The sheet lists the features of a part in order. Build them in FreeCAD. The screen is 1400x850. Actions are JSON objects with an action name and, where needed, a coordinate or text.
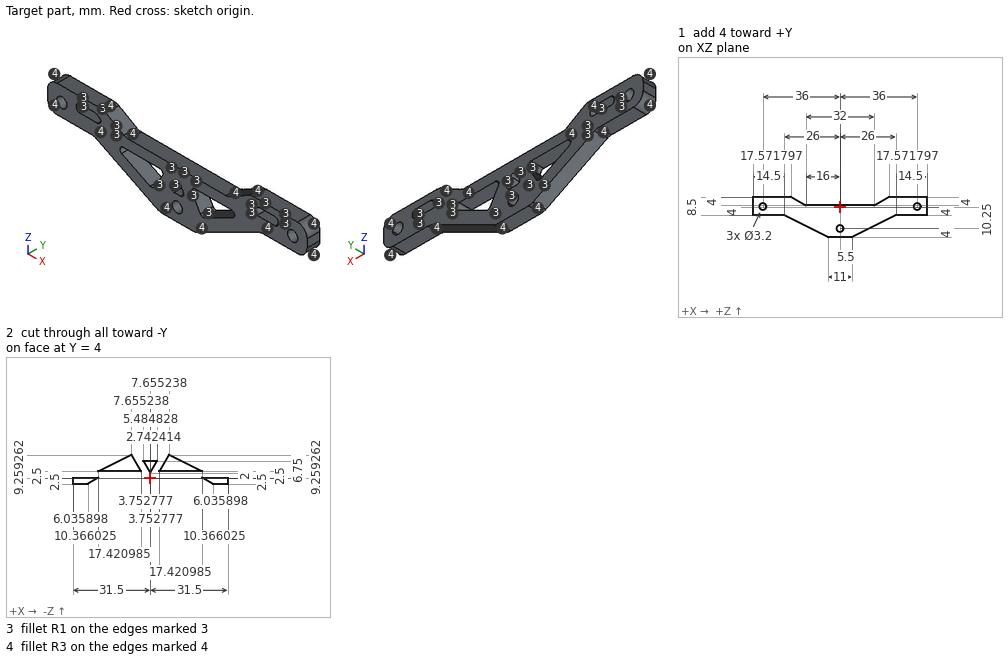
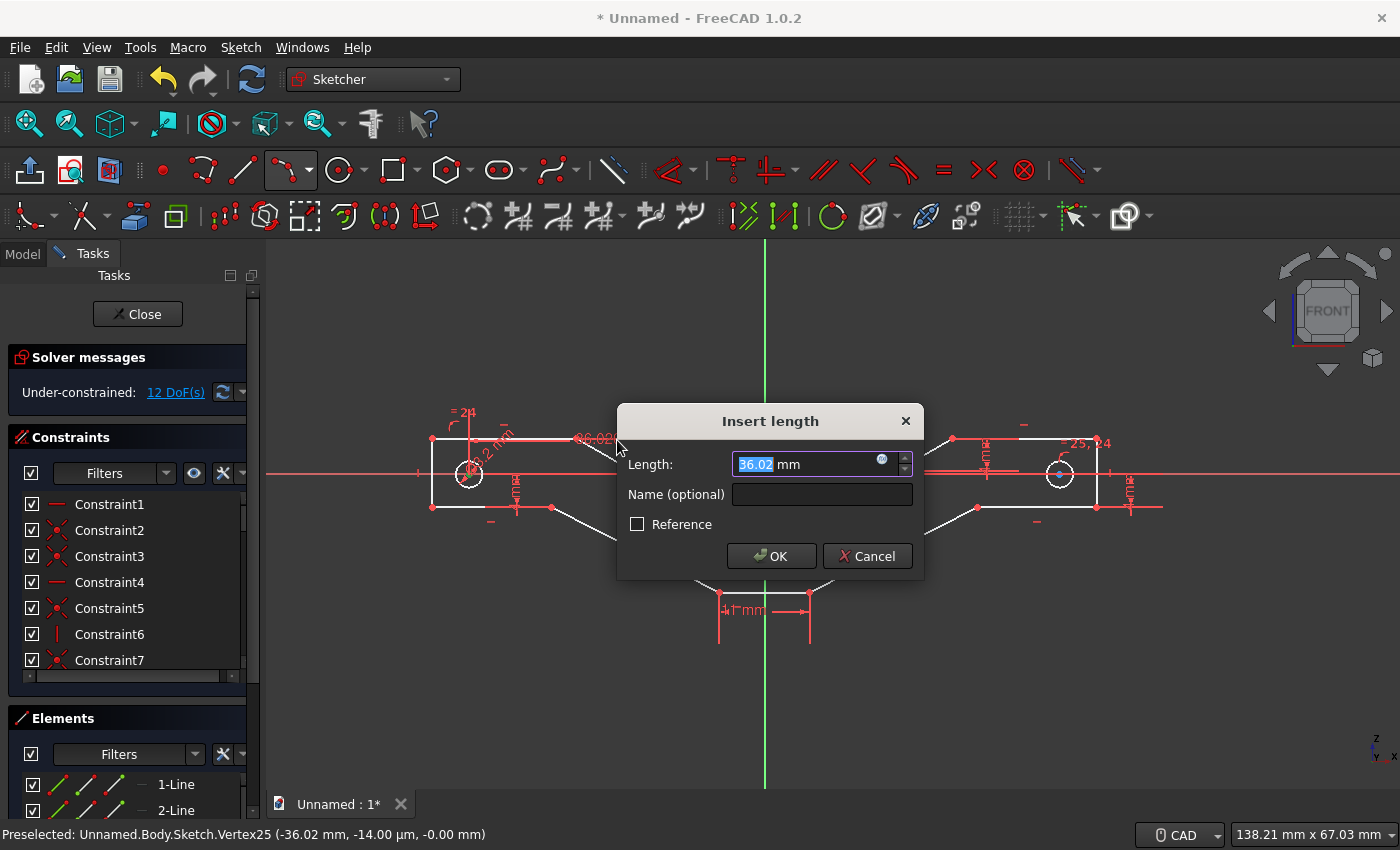
{"action": "type", "text": "36"}
{"action": "key", "text": "Return"}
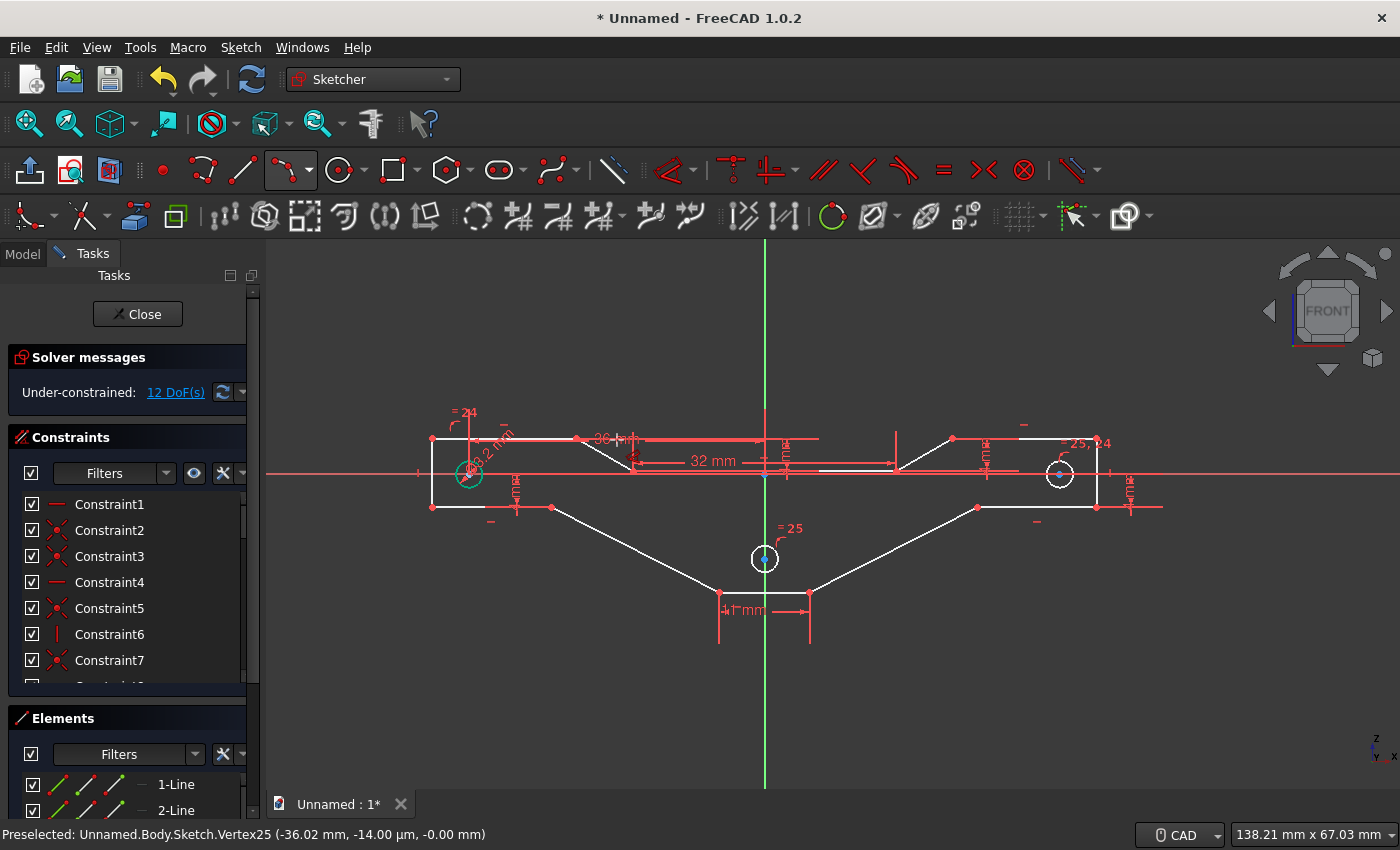
{"action": "left_click", "coordinate": [1060, 474]}
{"action": "left_click", "coordinate": [912, 440]}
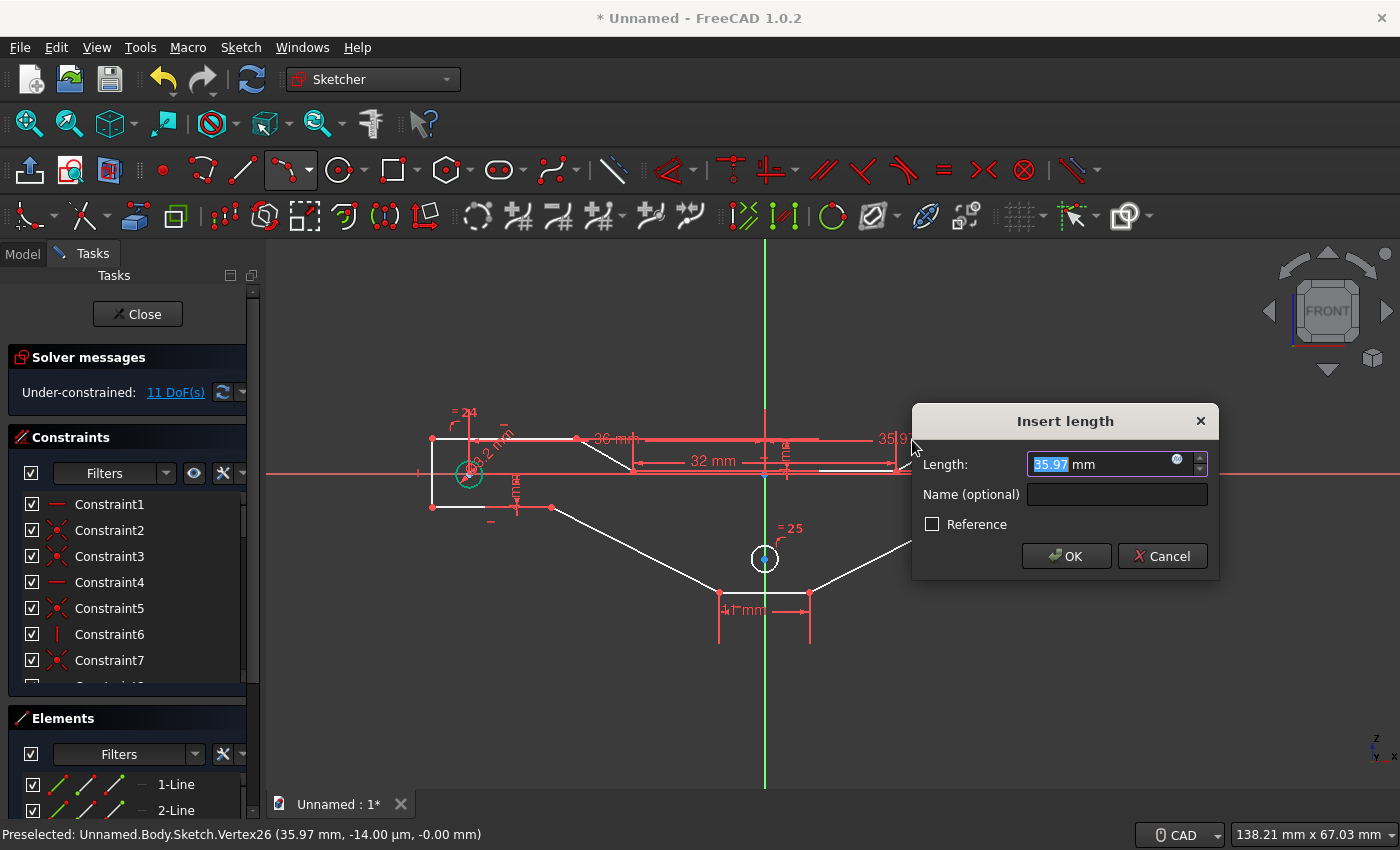
{"action": "type", "text": "36"}
{"action": "key", "text": "Return"}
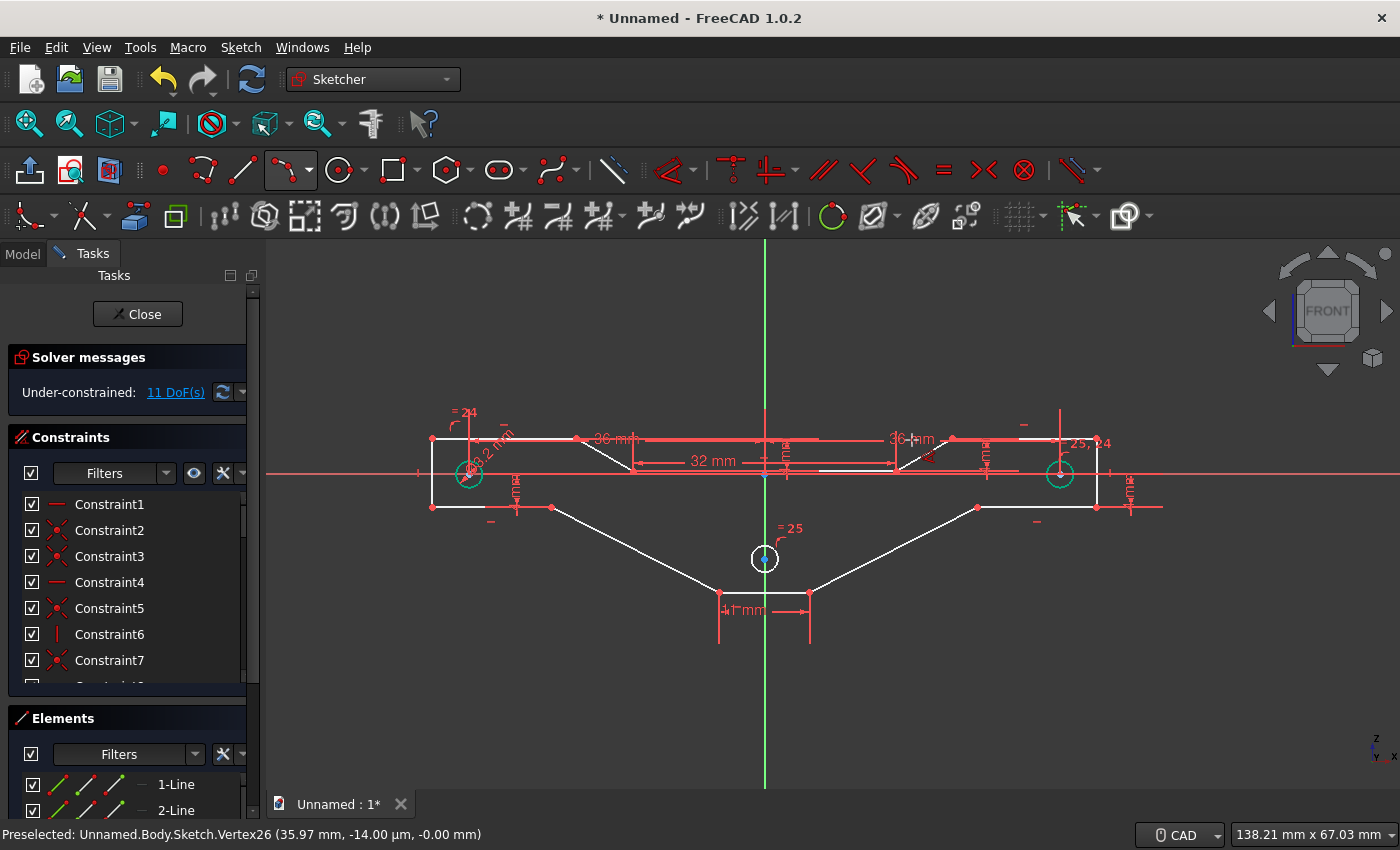
{"action": "left_click", "coordinate": [810, 593]}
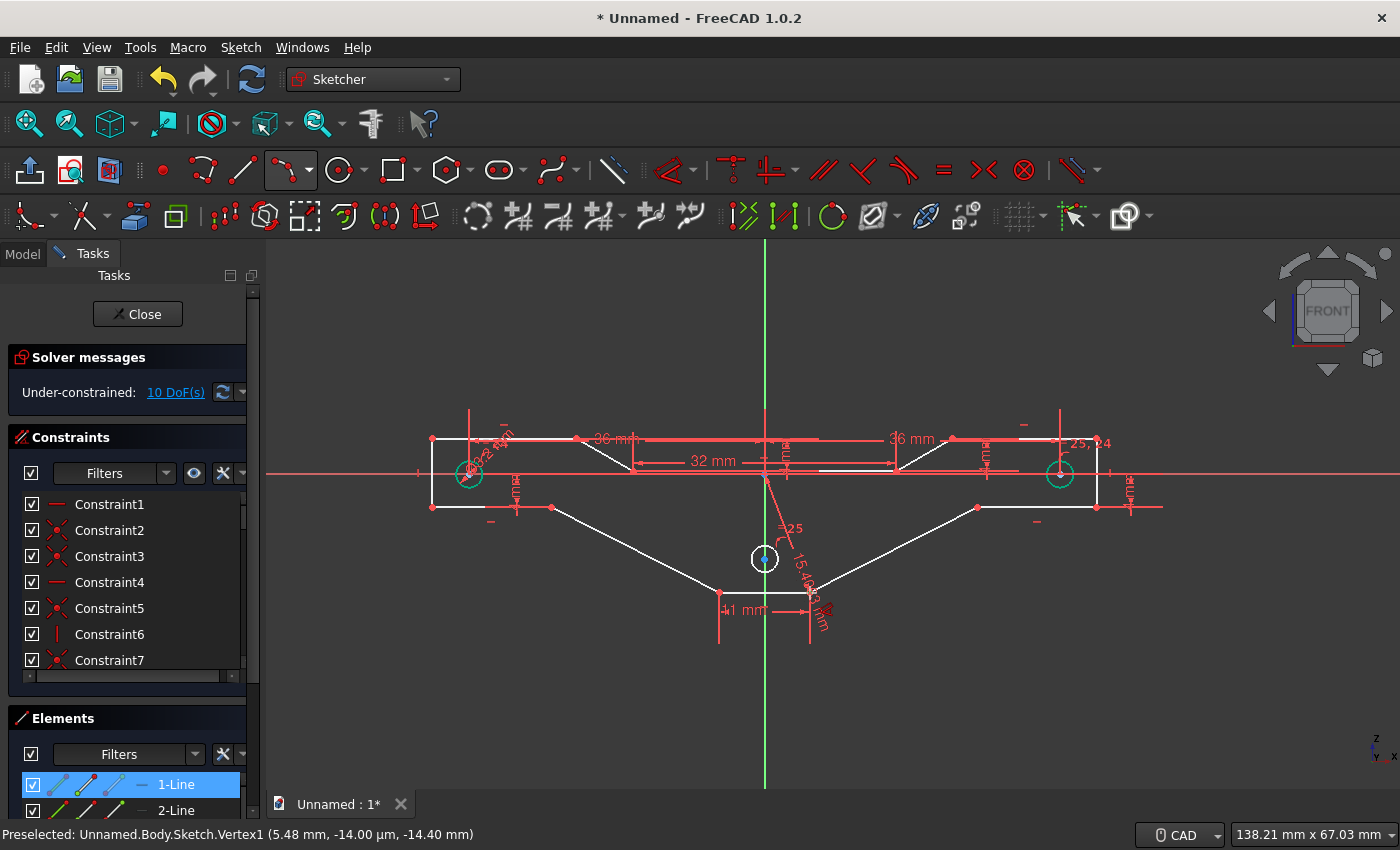
{"action": "left_click", "coordinate": [765, 559]}
{"action": "left_click", "coordinate": [731, 576]}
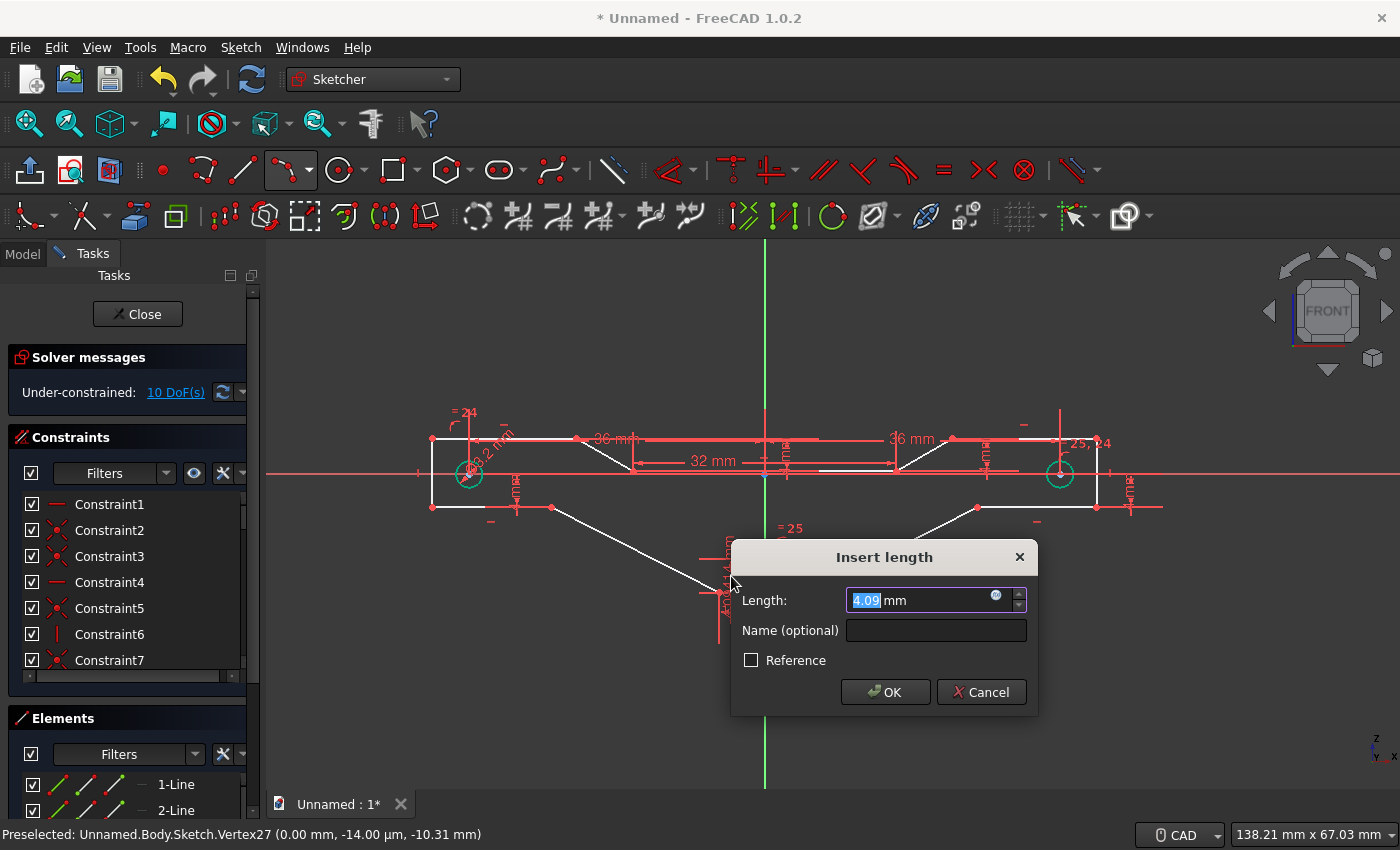
{"action": "type", "text": "4"}
{"action": "key", "text": "Return"}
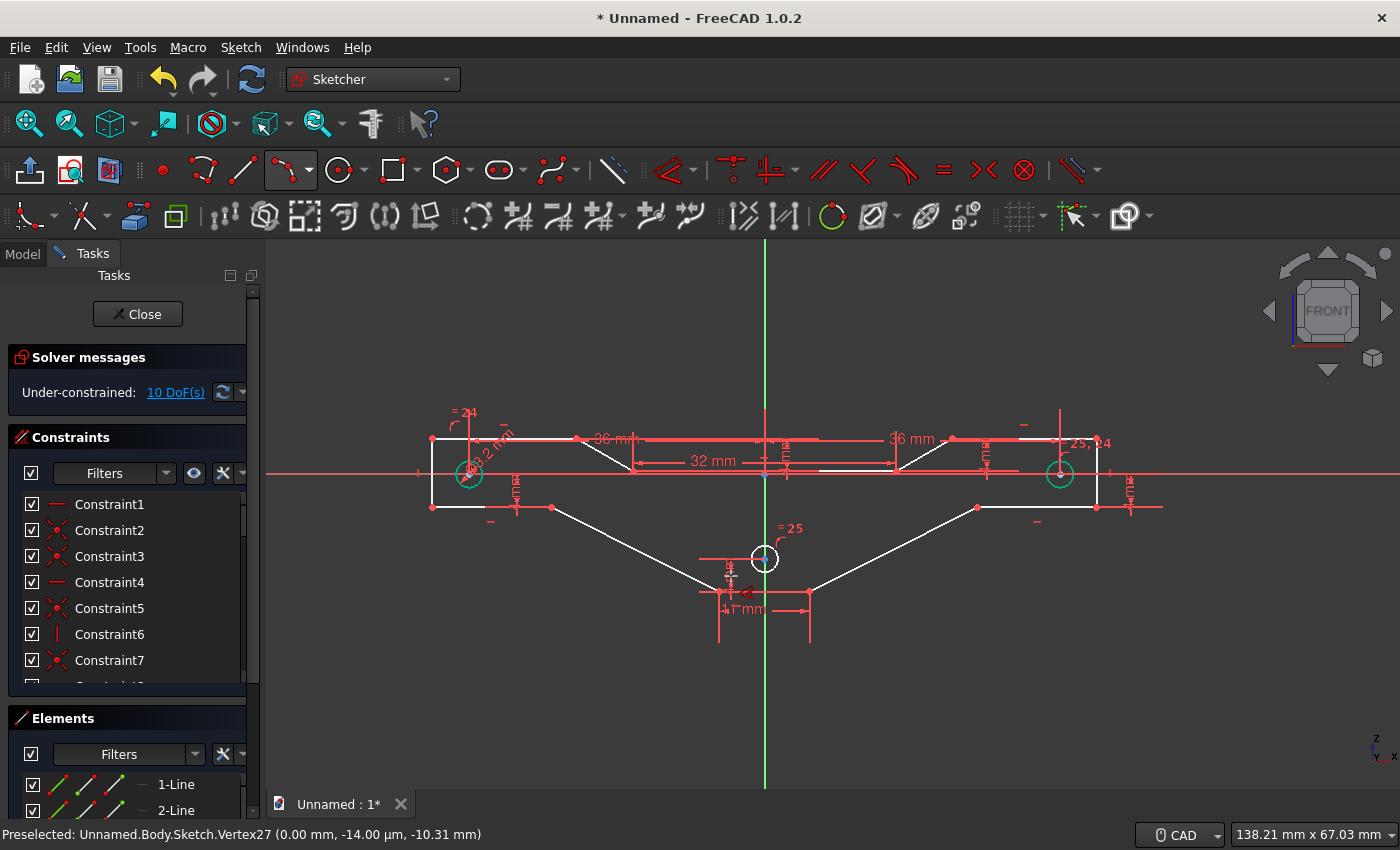
{"action": "left_click", "coordinate": [432, 487]}
{"action": "left_click", "coordinate": [398, 457]}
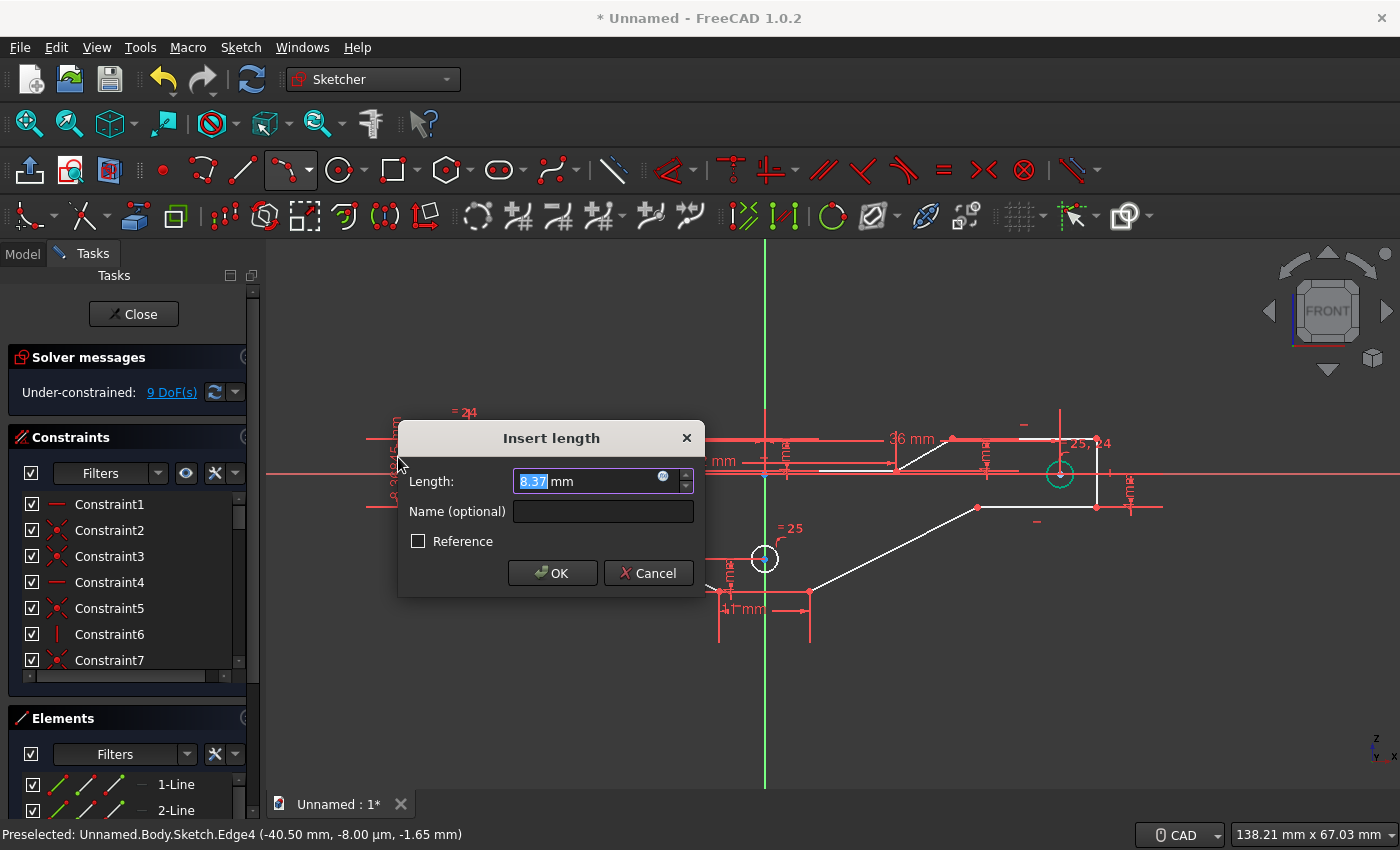
{"action": "type", "text": "8.5"}
{"action": "key", "text": "Return"}